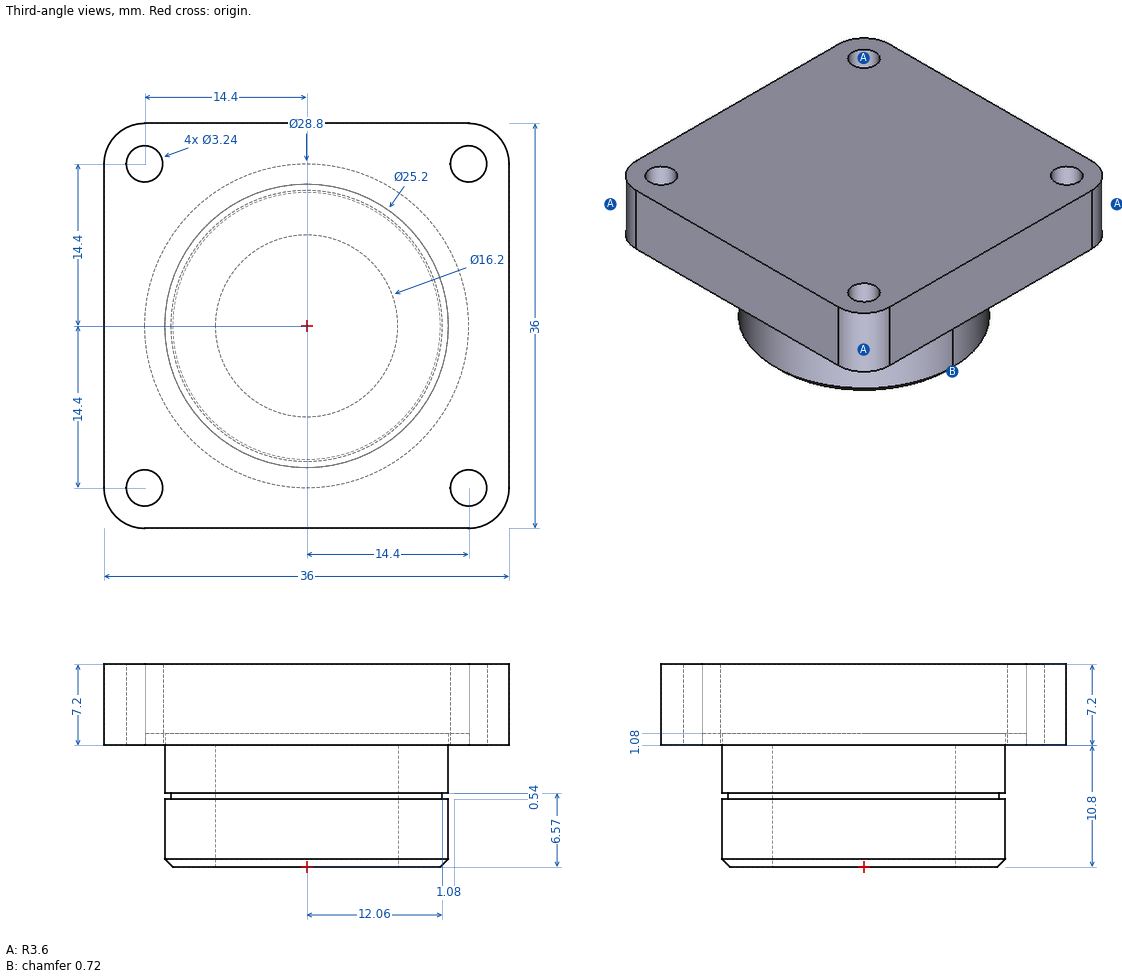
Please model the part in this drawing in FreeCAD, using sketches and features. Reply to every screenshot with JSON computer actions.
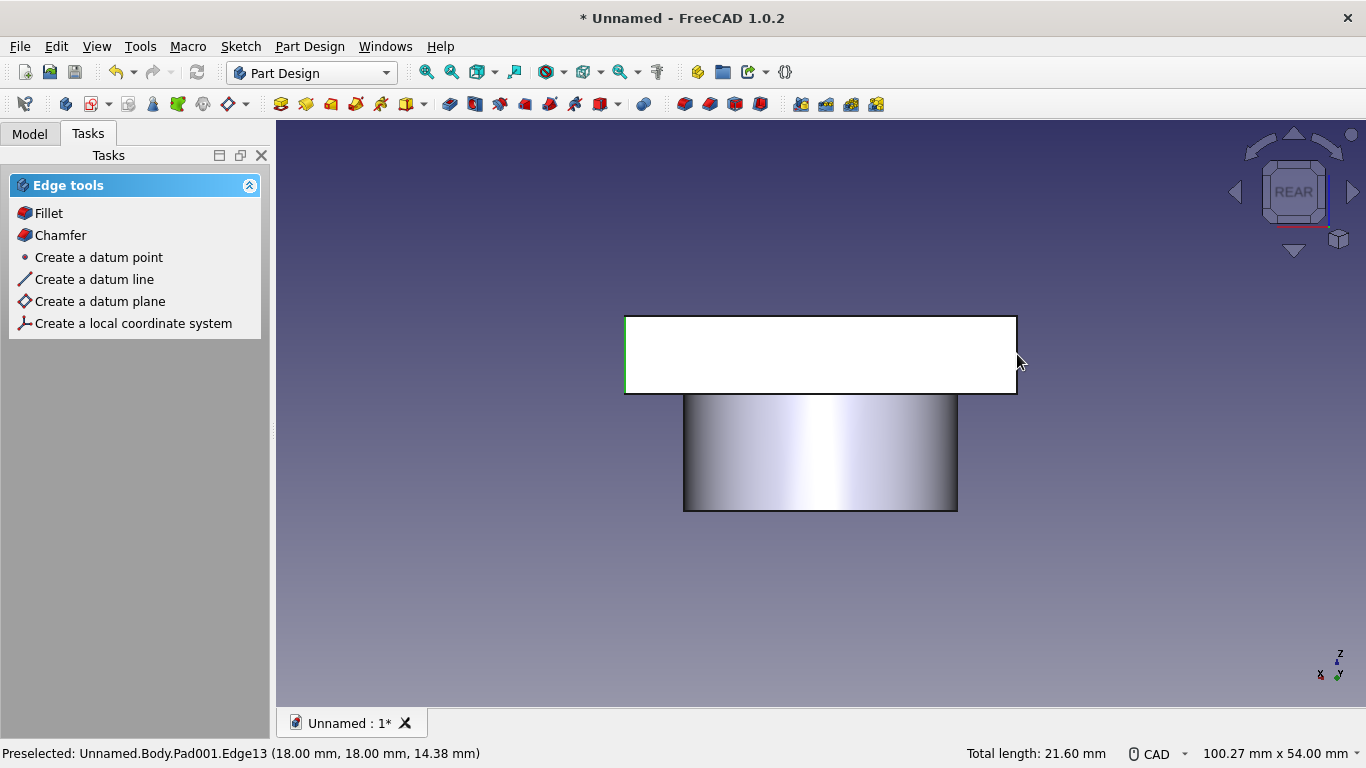
{"action": "key", "text": "v f"}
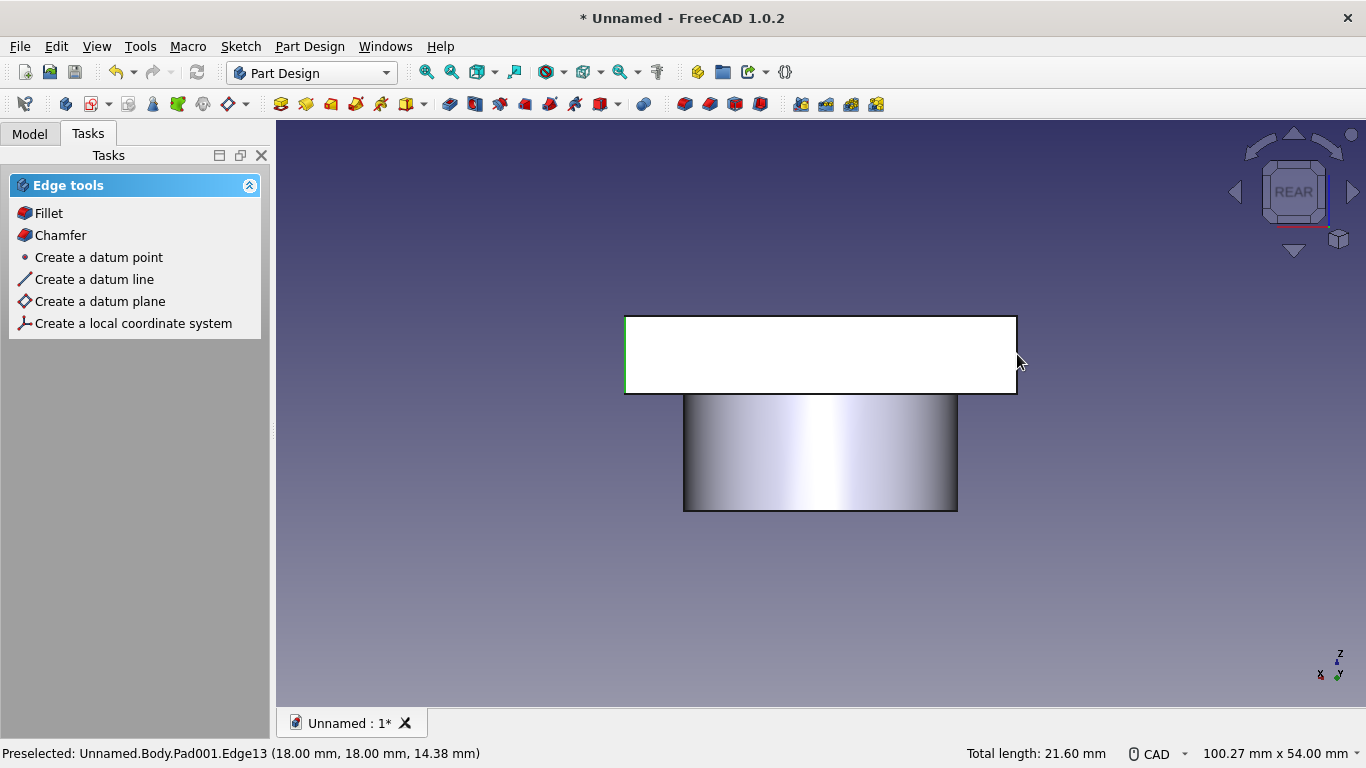
{"action": "left_click", "coordinate": [1017, 354], "text": "ctrl"}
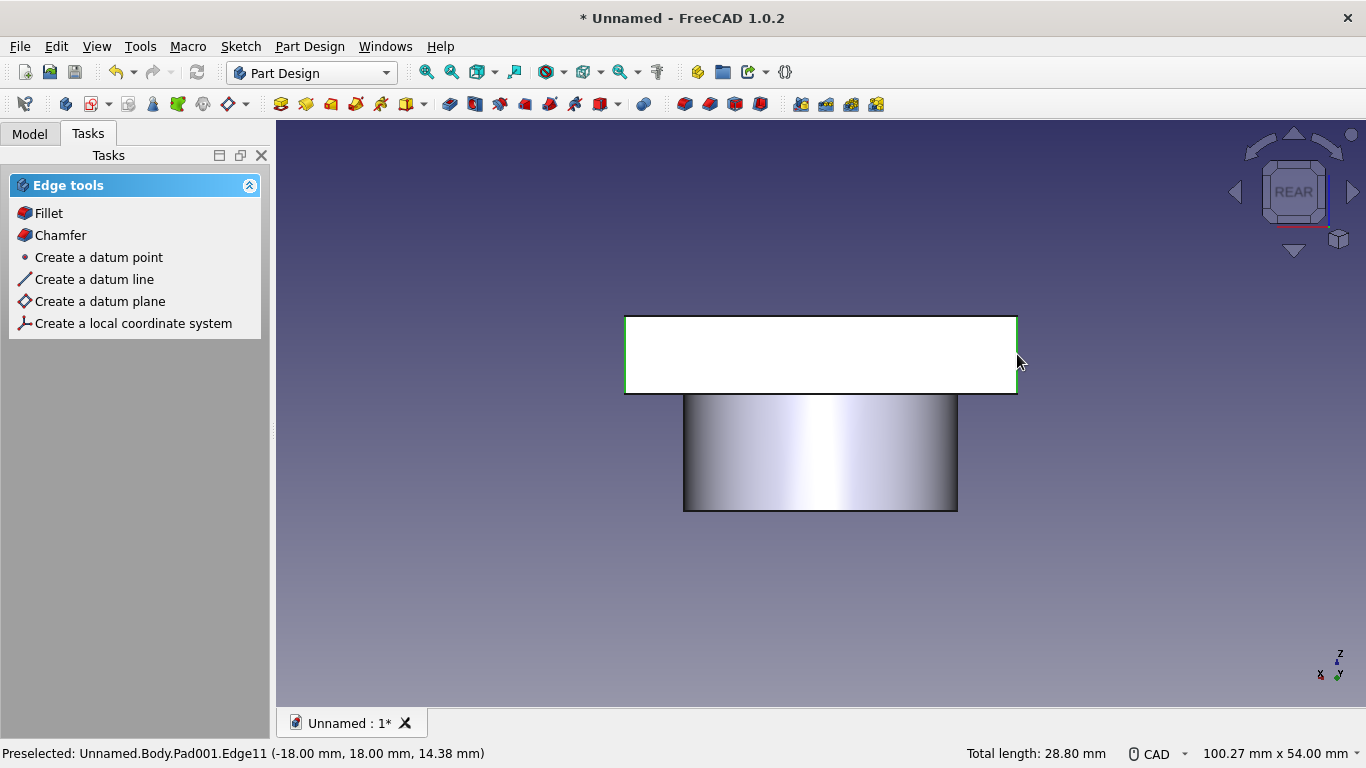
{"action": "left_click", "coordinate": [685, 104]}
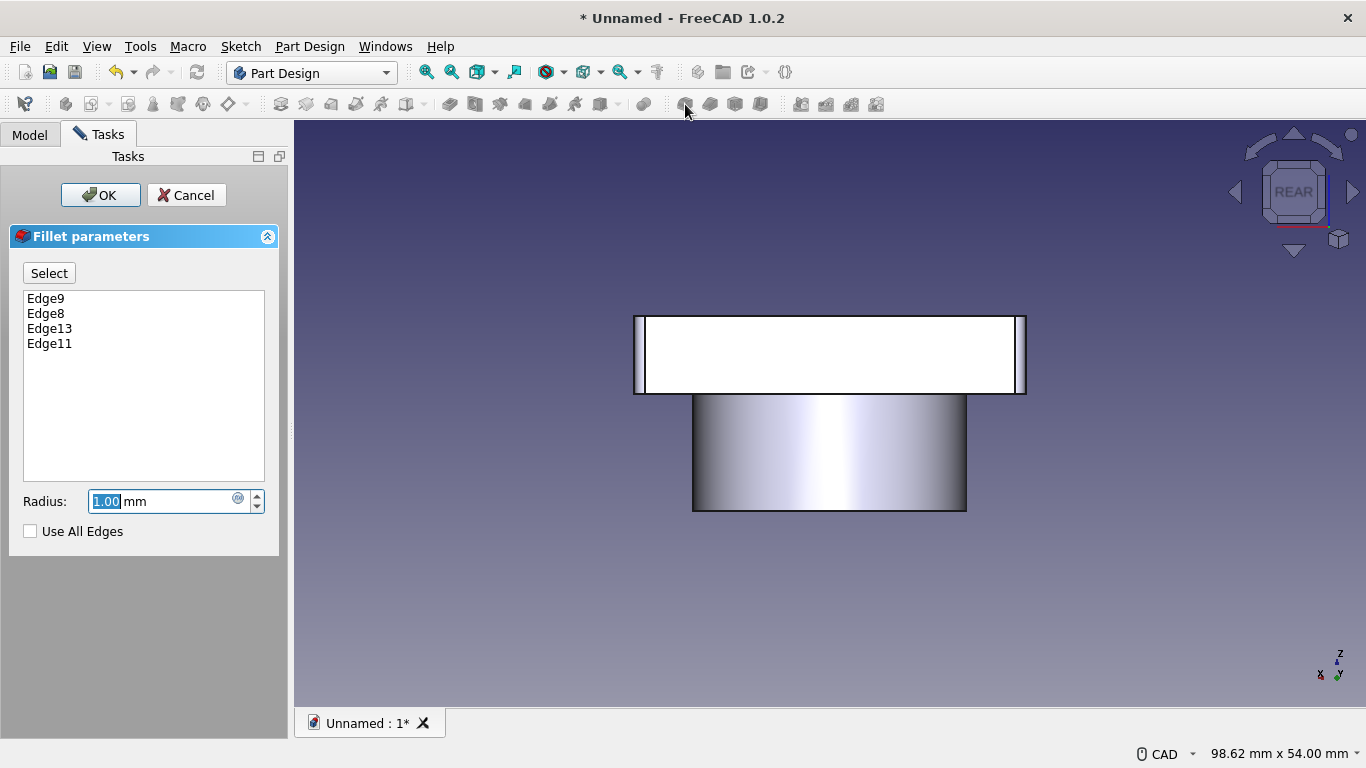
{"action": "type", "text": "3.6"}
{"action": "key", "text": "Tab"}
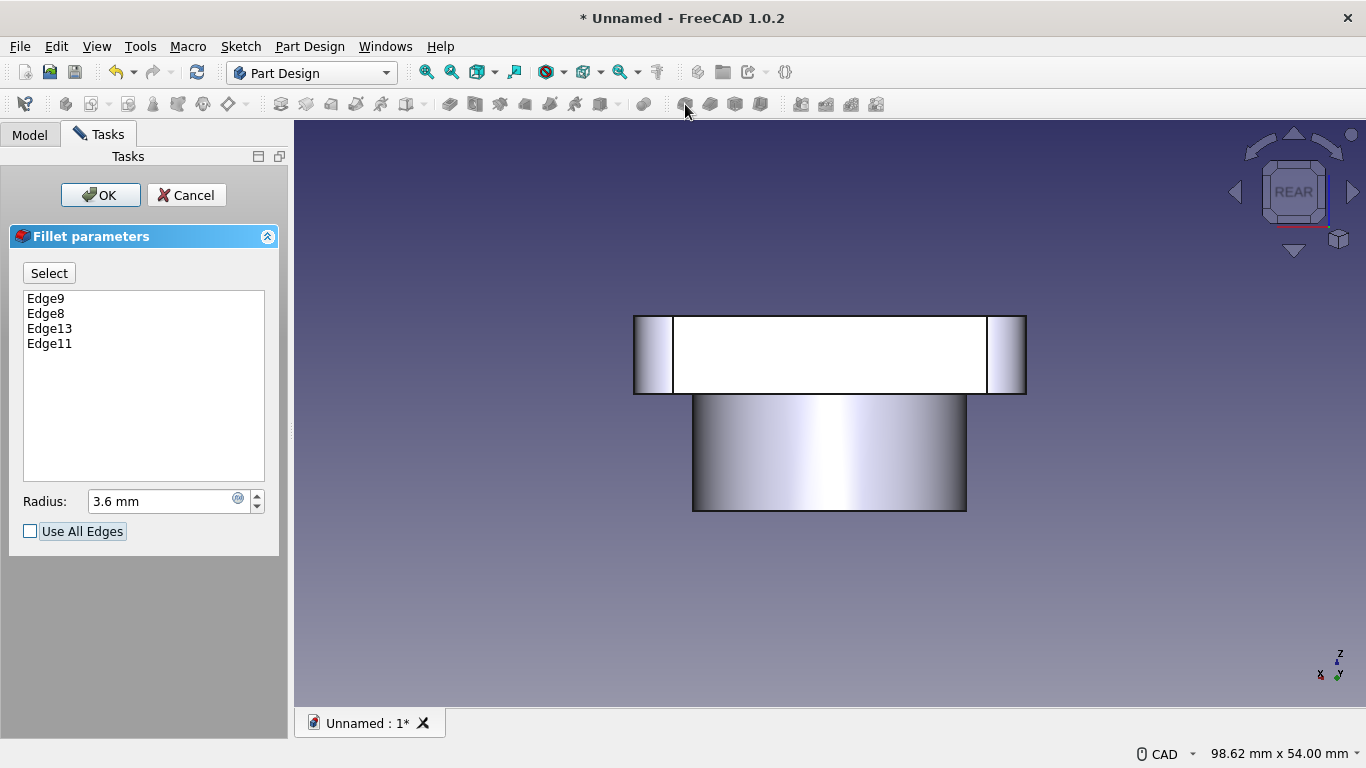
{"action": "left_click", "coordinate": [101, 195]}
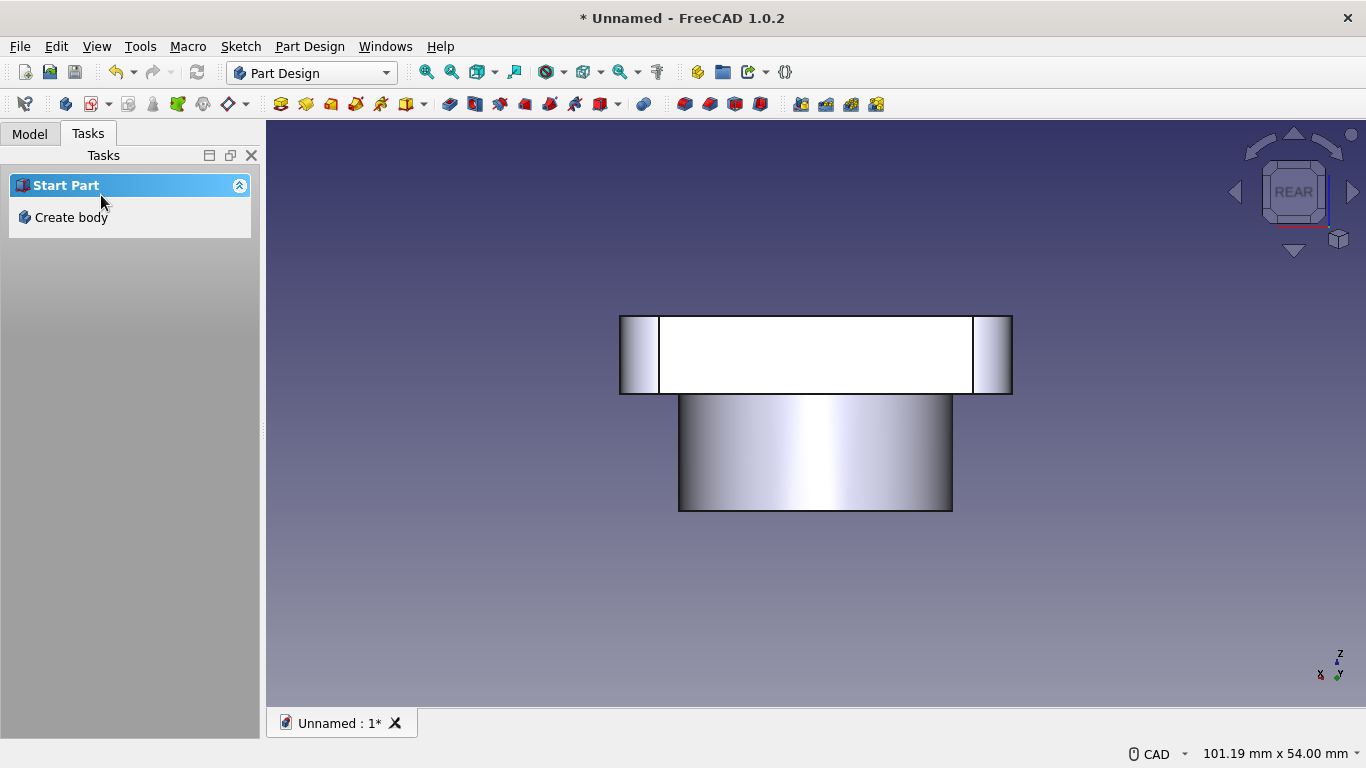
{"action": "key", "text": "v f"}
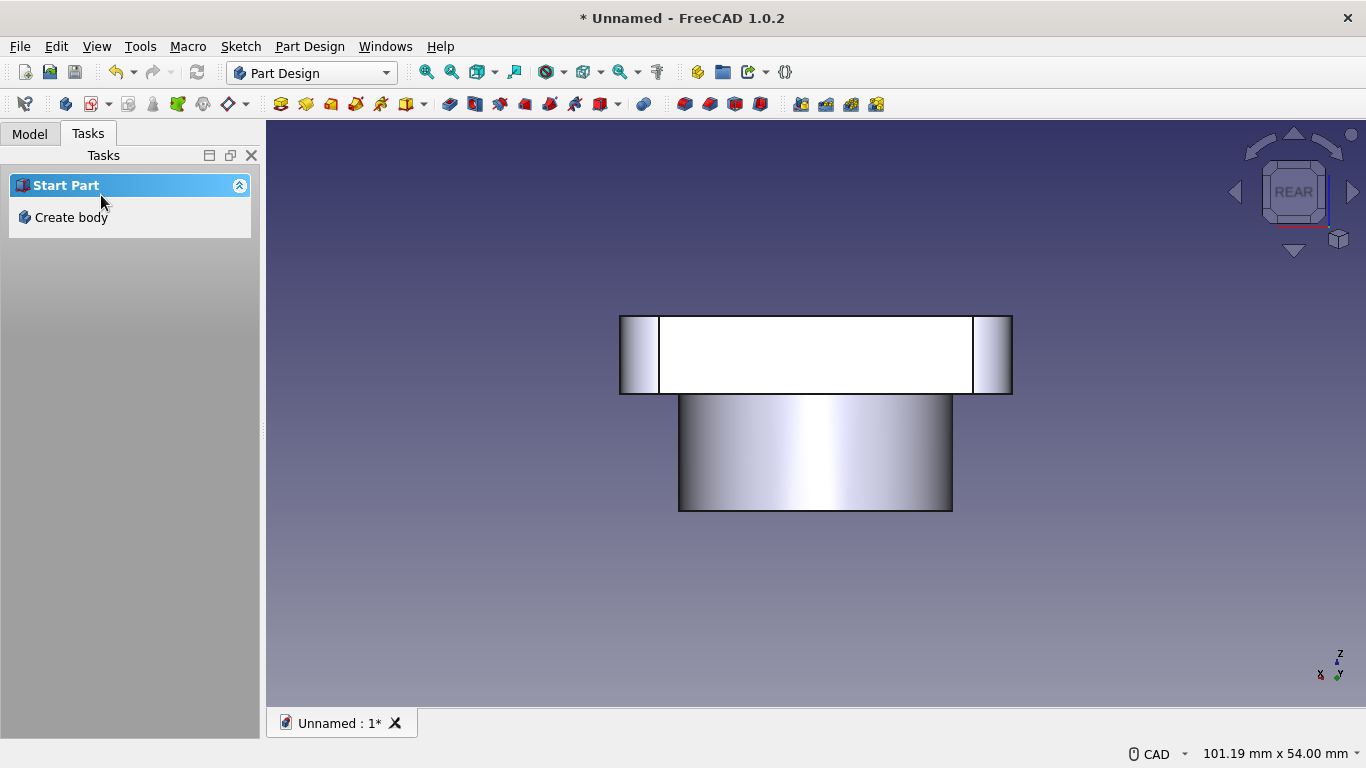
{"action": "key", "text": "0"}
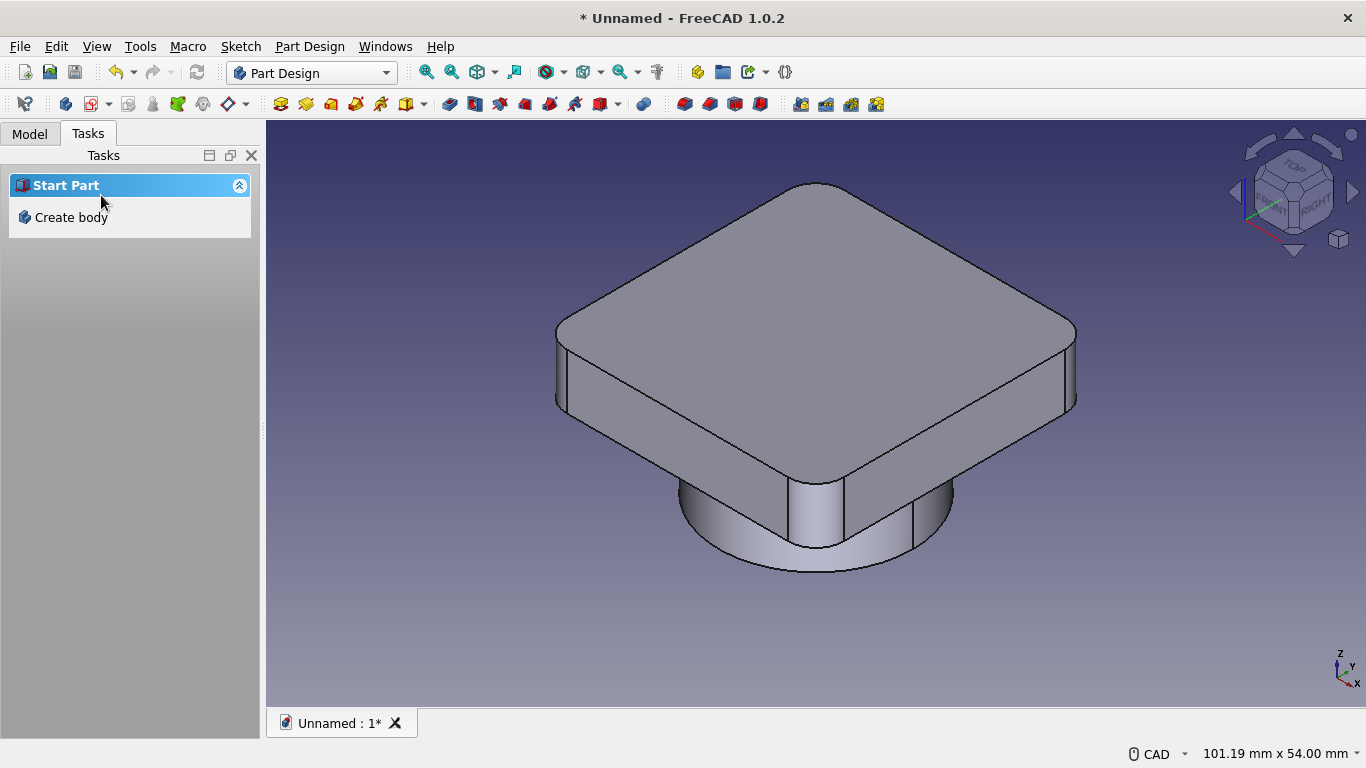
{"action": "key", "text": "2"}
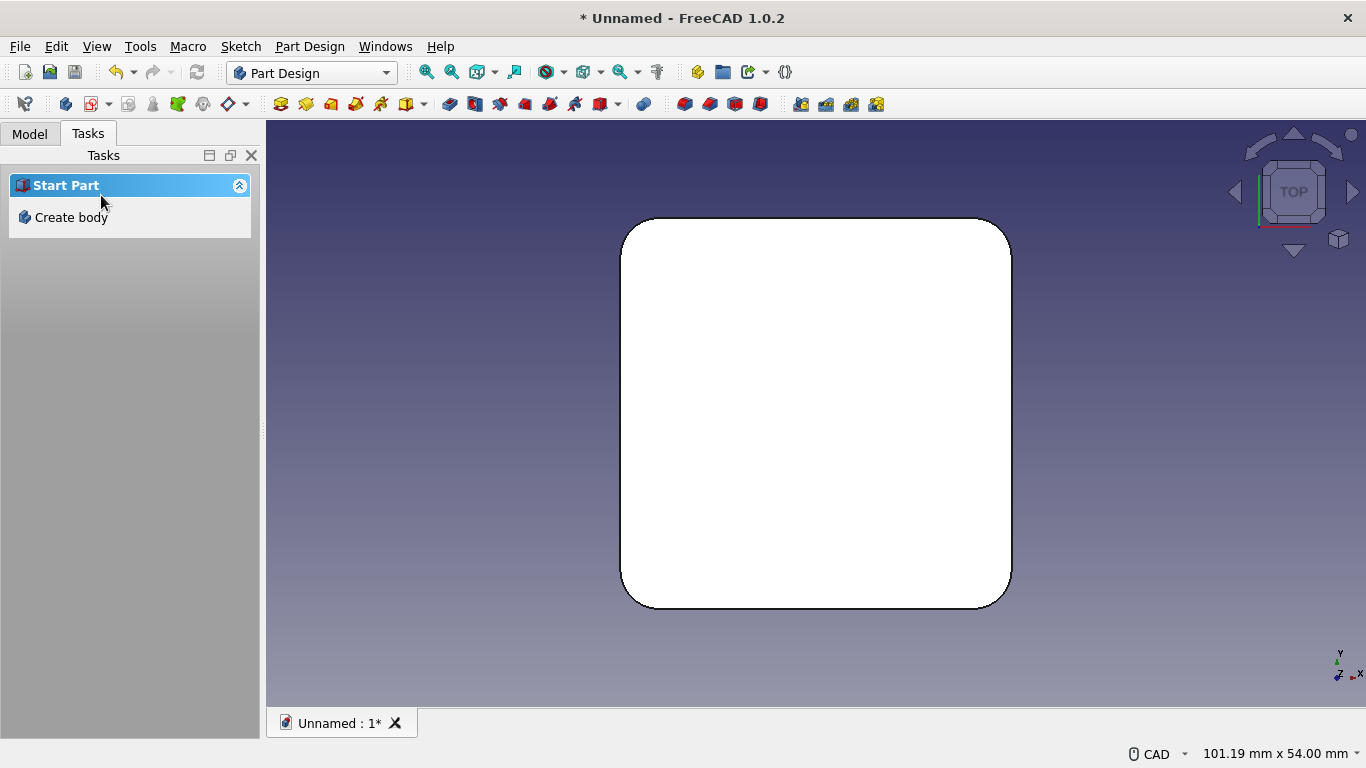
{"action": "key", "text": "1"}